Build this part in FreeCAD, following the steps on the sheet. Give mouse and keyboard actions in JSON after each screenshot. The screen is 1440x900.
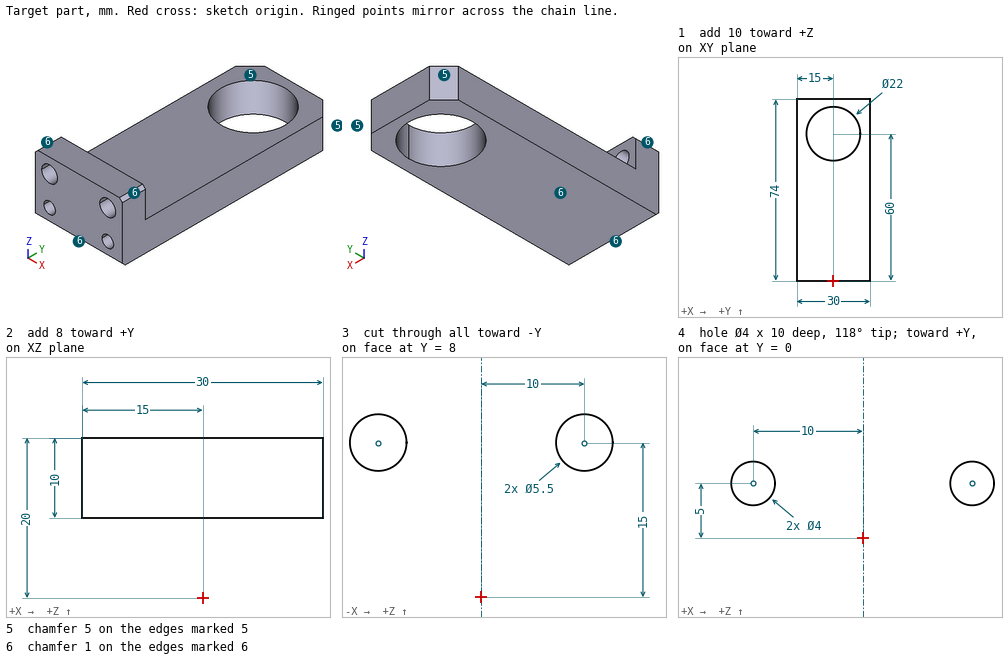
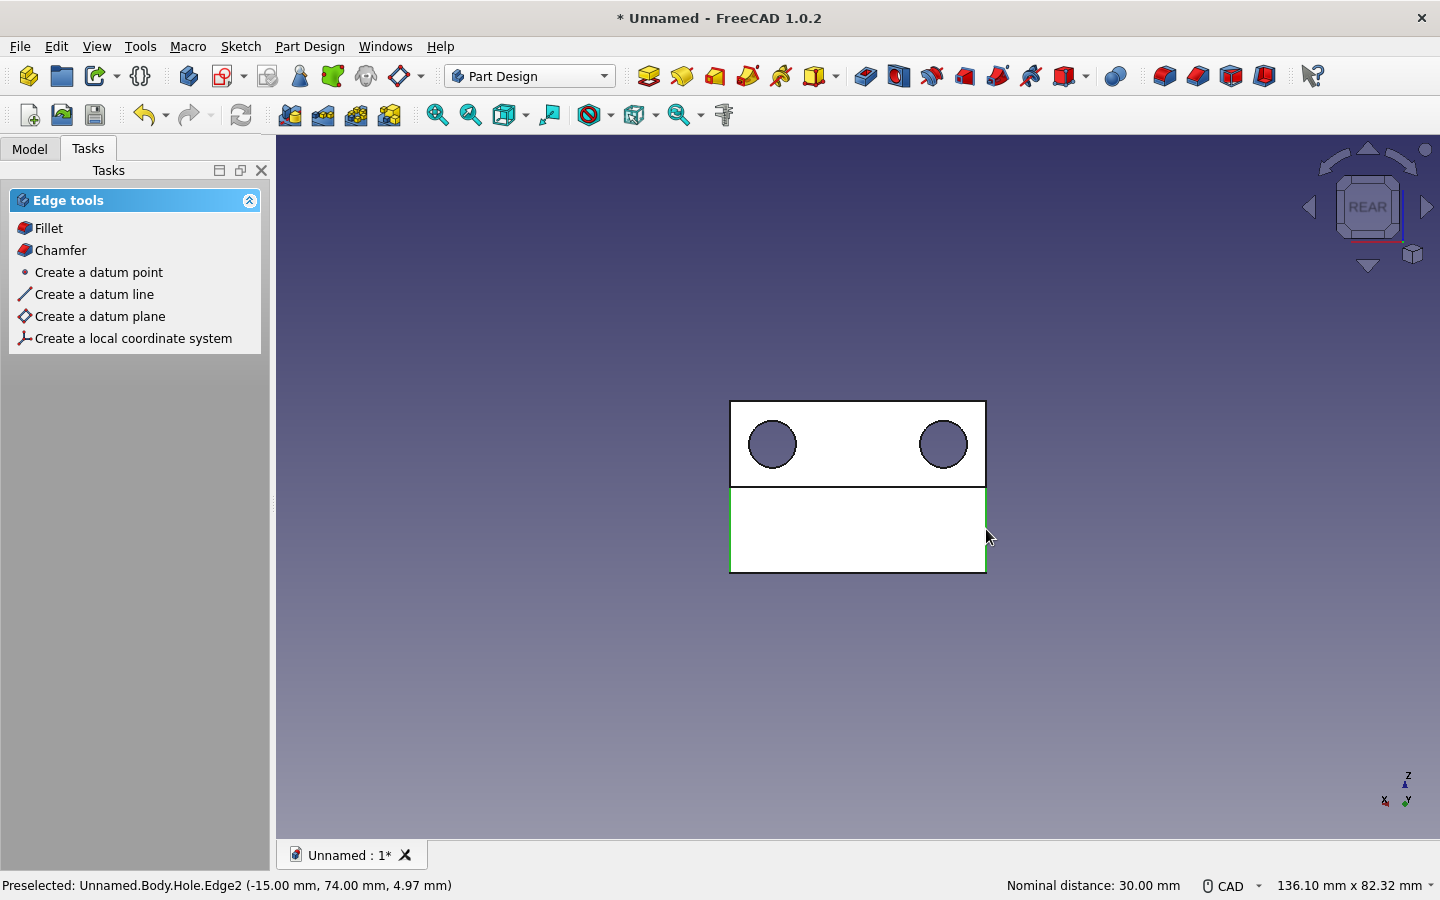
{"action": "left_click", "coordinate": [1198, 76]}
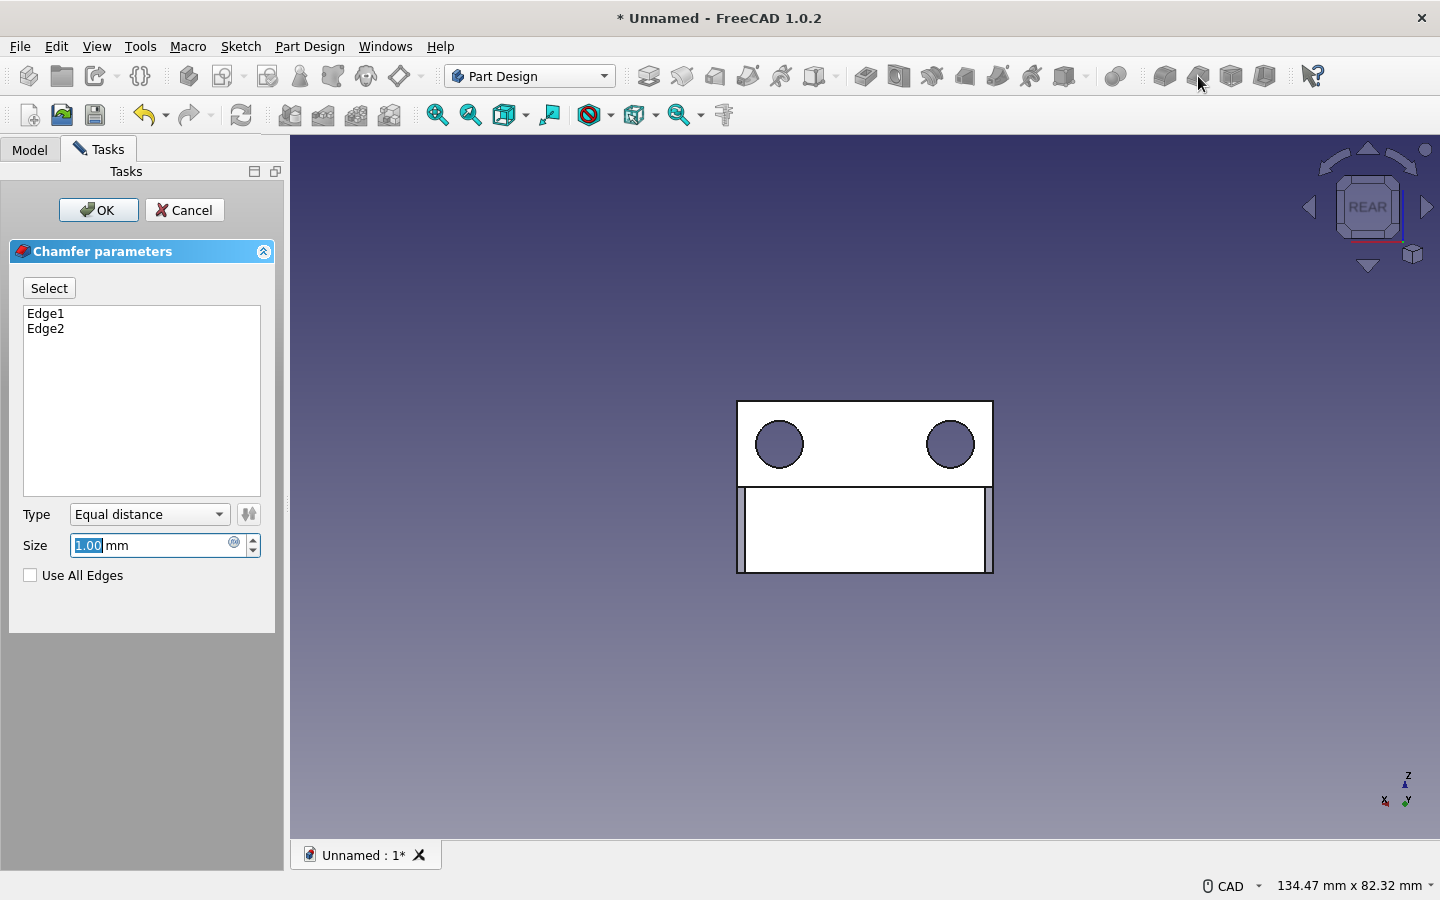
{"action": "type", "text": "5"}
{"action": "key", "text": "Tab"}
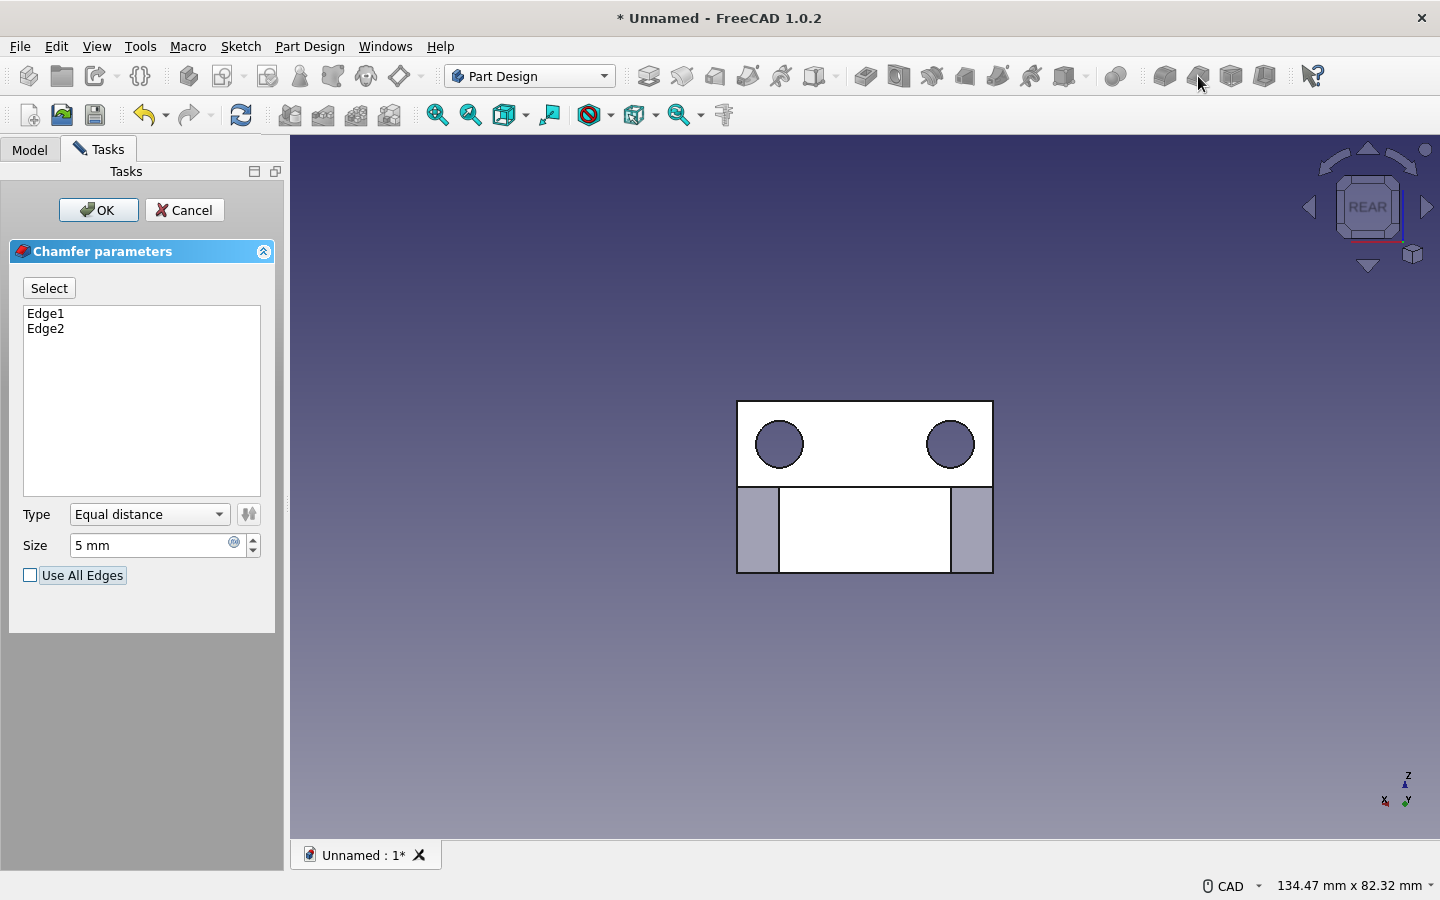
{"action": "left_click", "coordinate": [99, 210]}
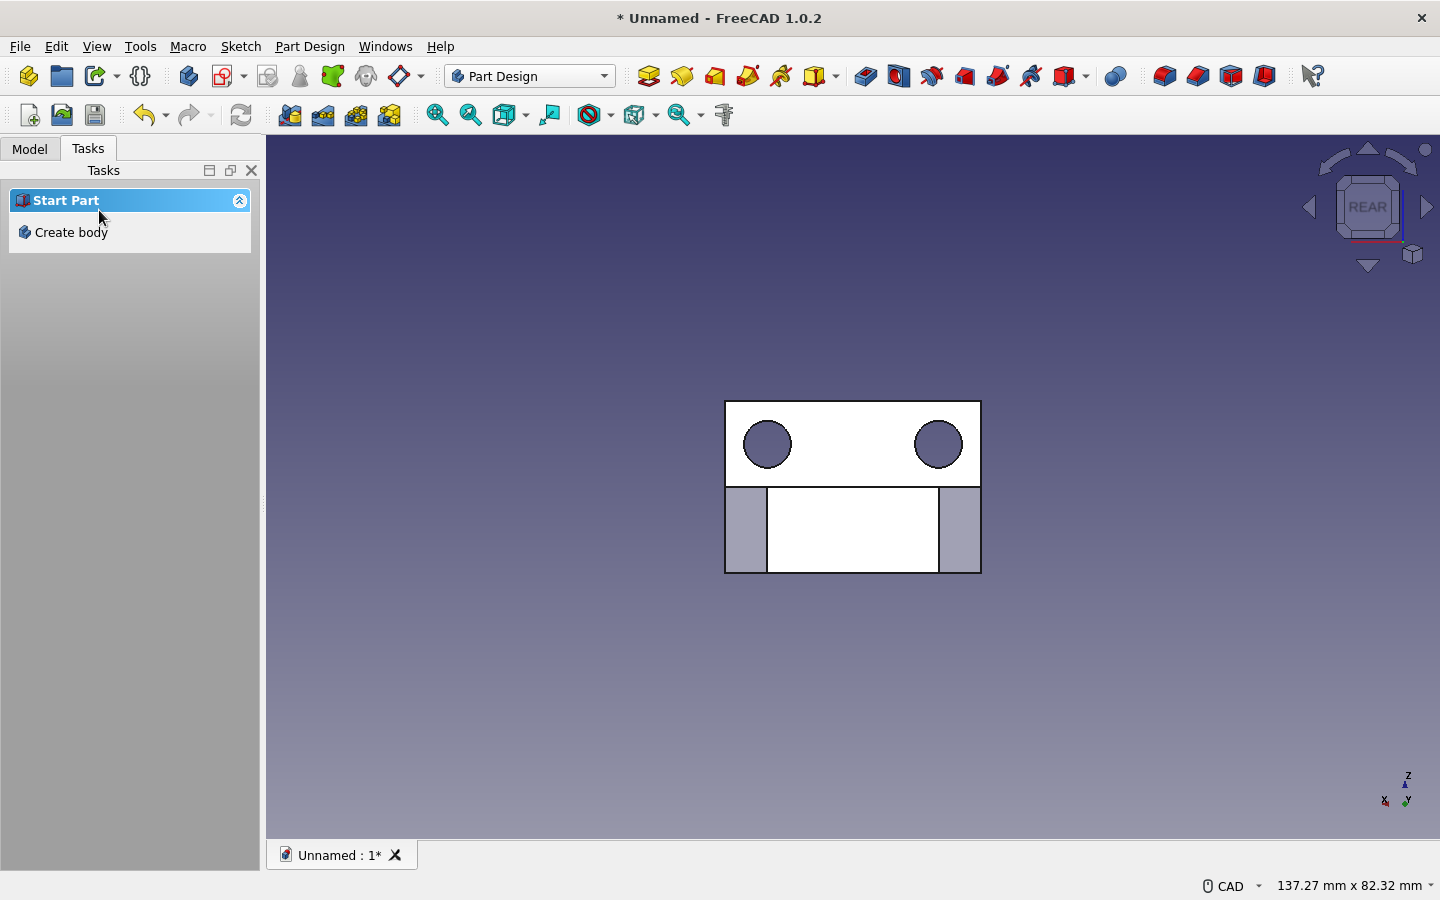
{"action": "left_click", "coordinate": [438, 116]}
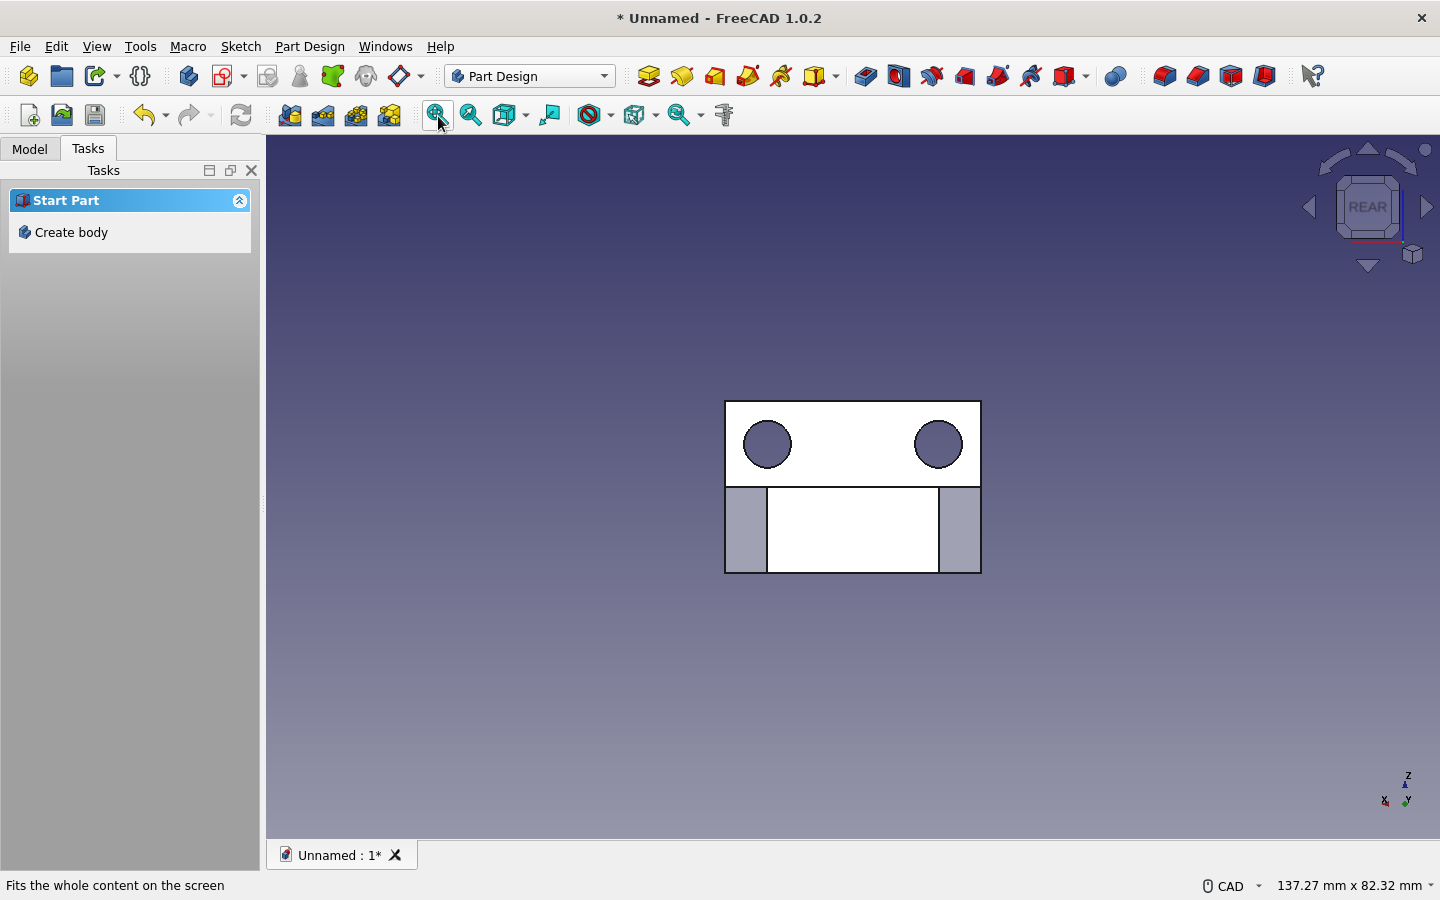
{"action": "key", "text": "0"}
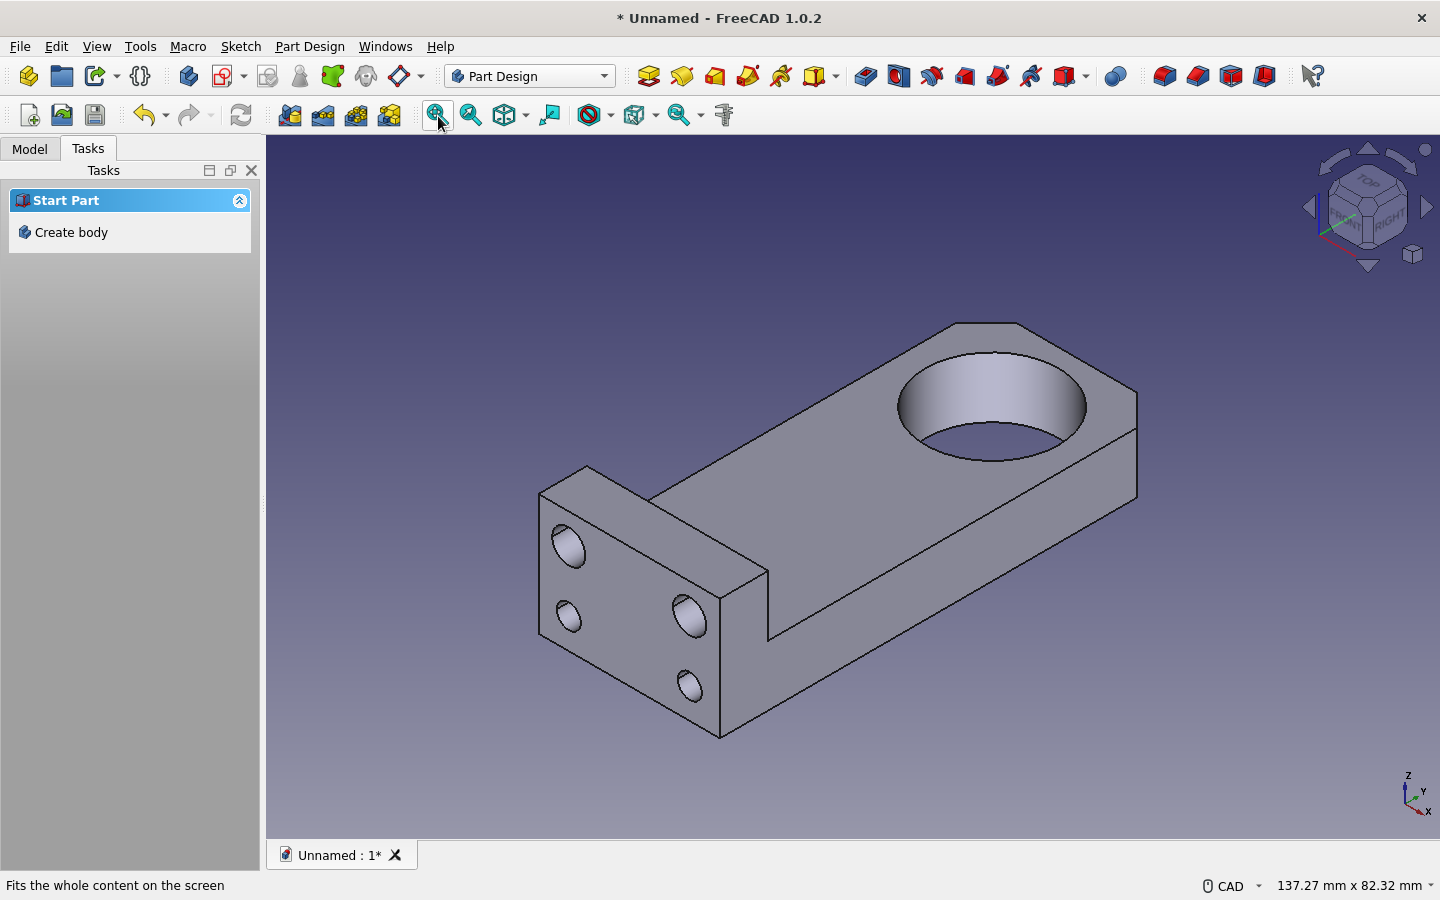
{"action": "left_click", "coordinate": [744, 584]}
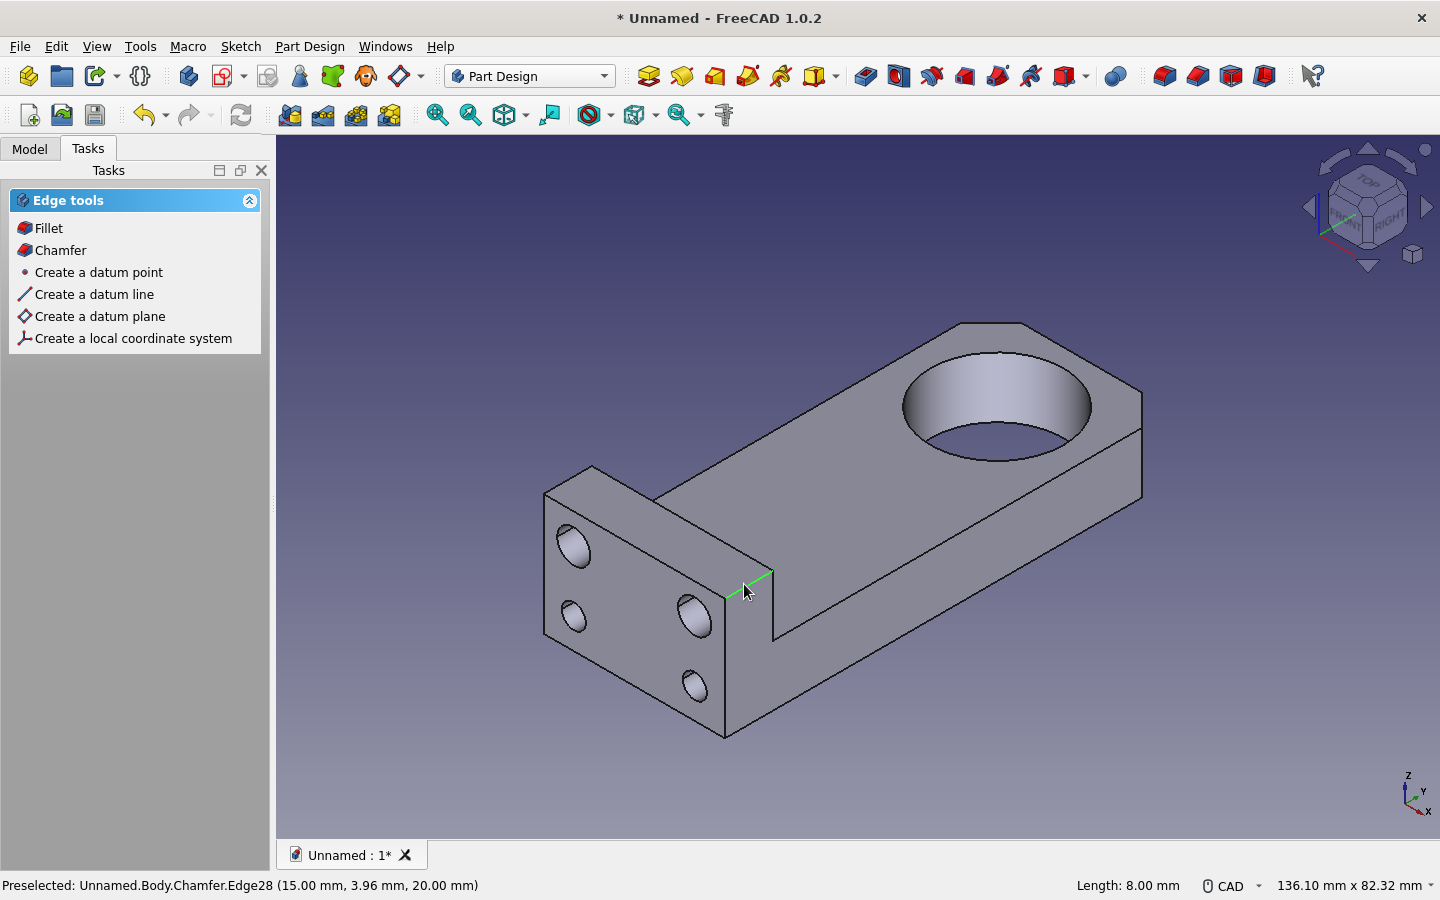
{"action": "key", "text": "2"}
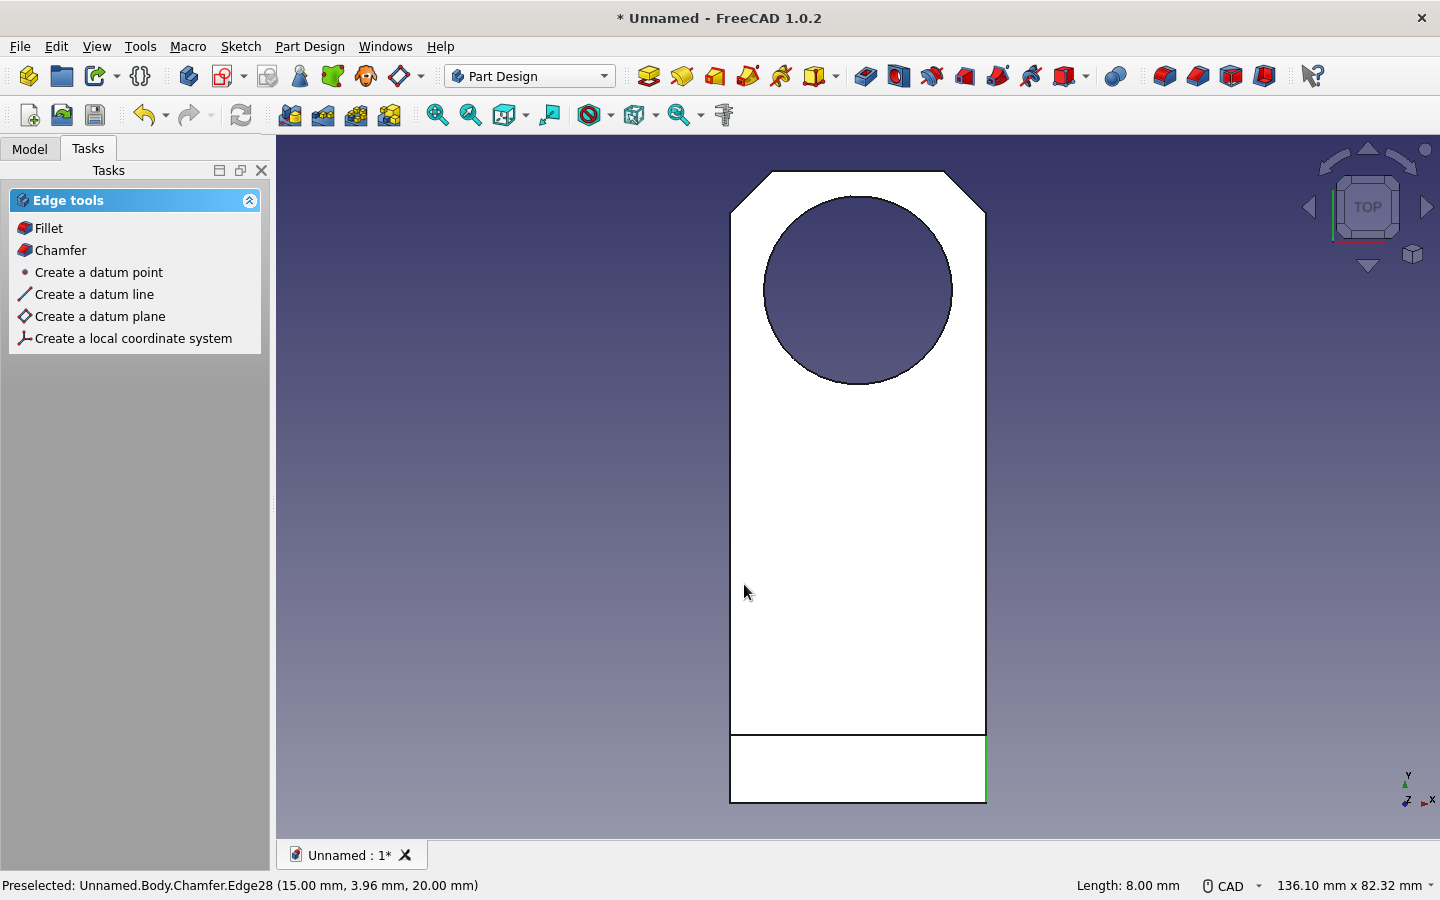
{"action": "left_click", "coordinate": [730, 768], "text": "ctrl"}